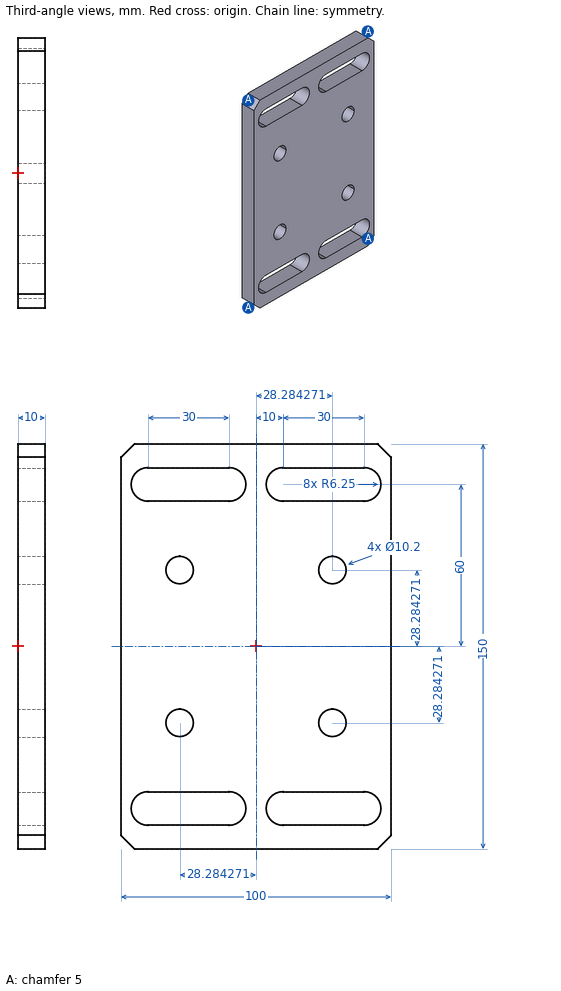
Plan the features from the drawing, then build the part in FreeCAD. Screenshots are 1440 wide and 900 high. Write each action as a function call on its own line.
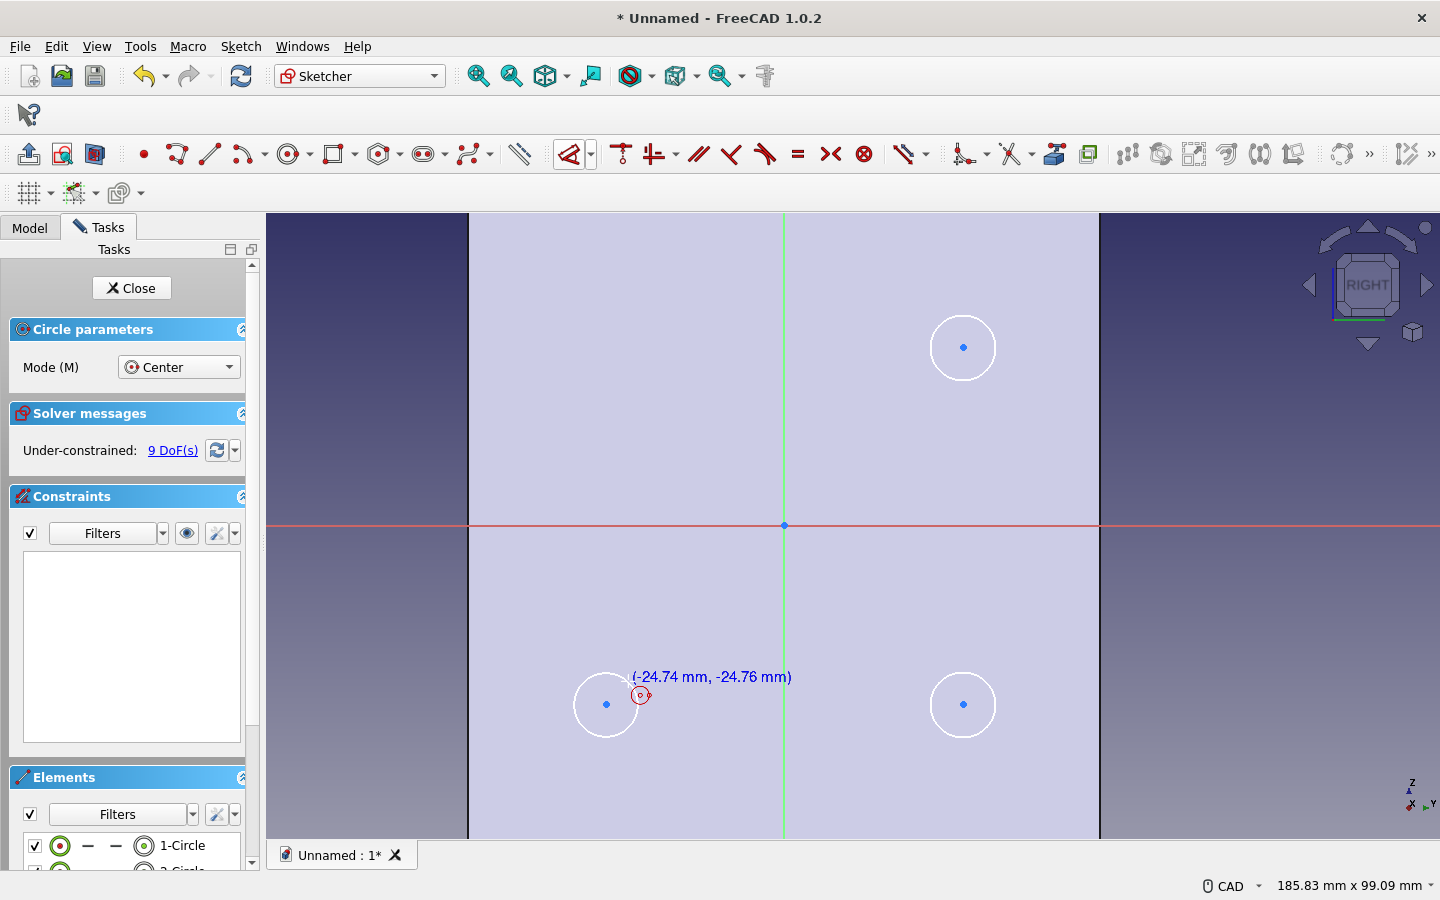
click(606, 347)
click(628, 324)
key(Escape)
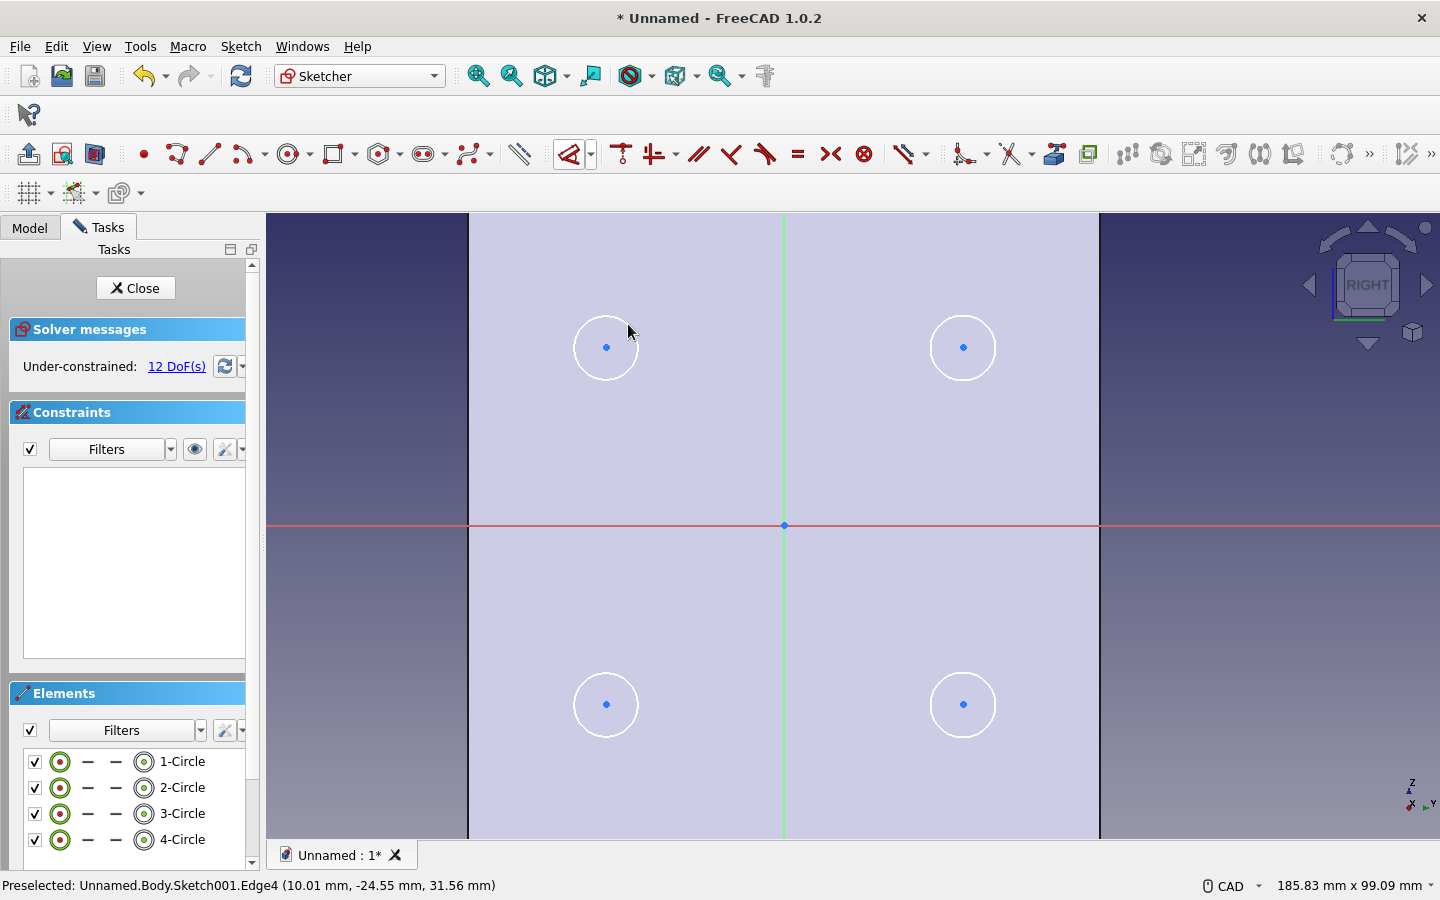
click(986, 325)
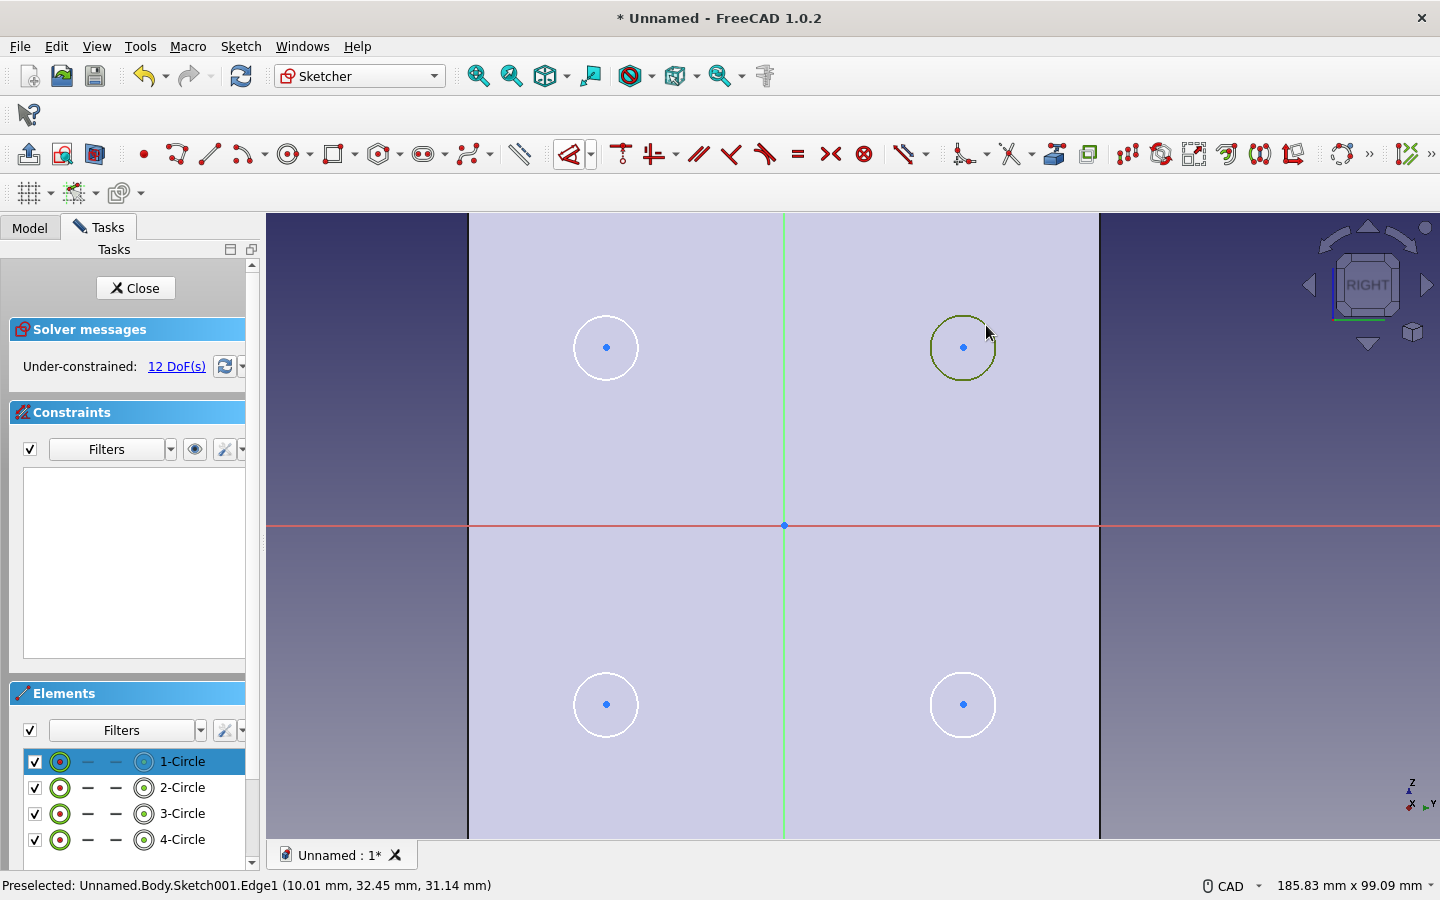
click(986, 682)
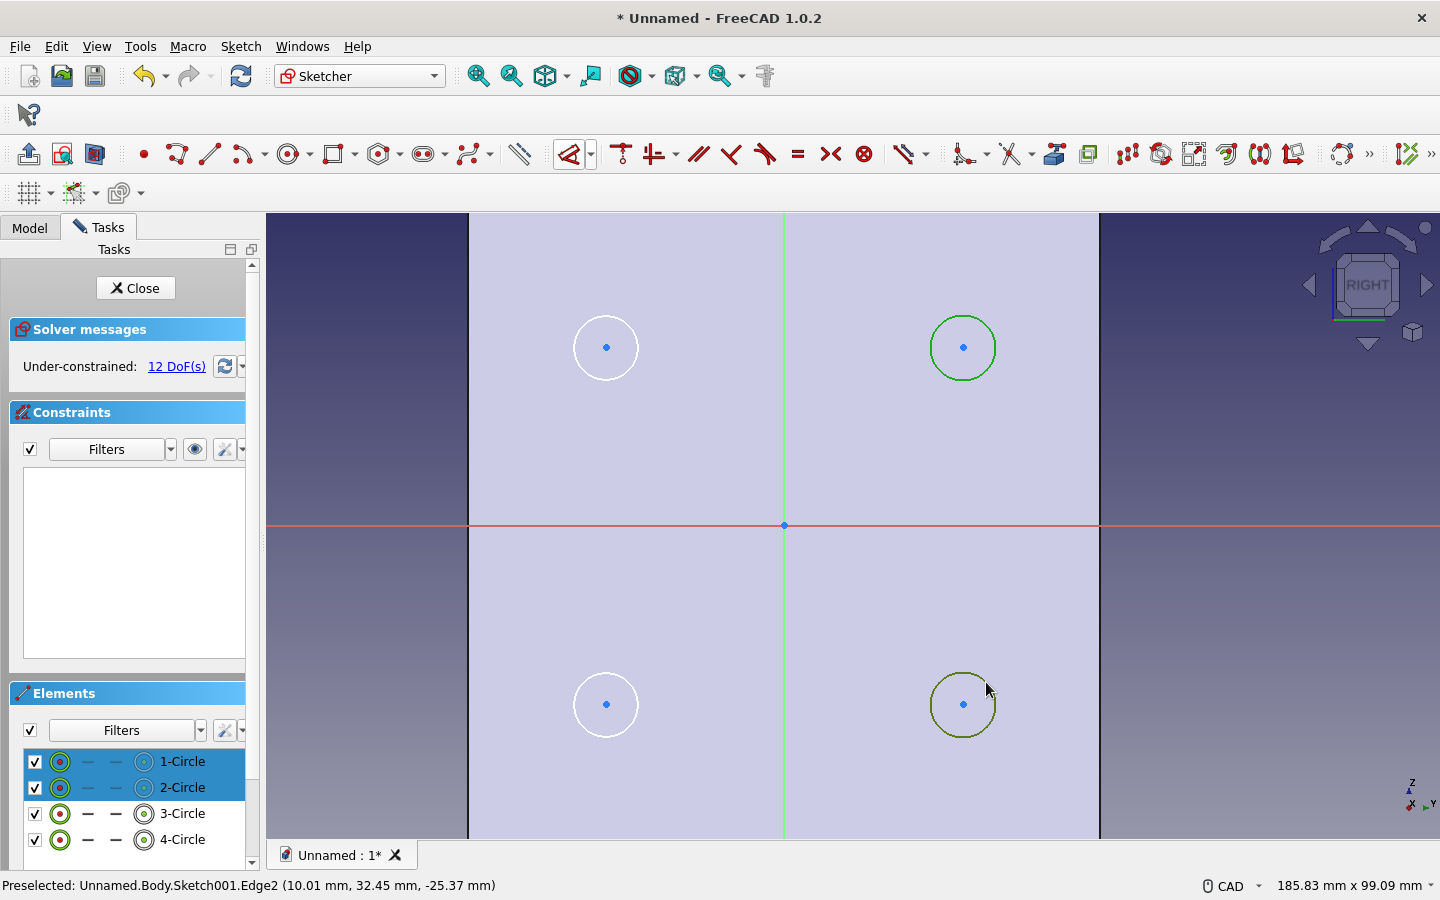
click(628, 682)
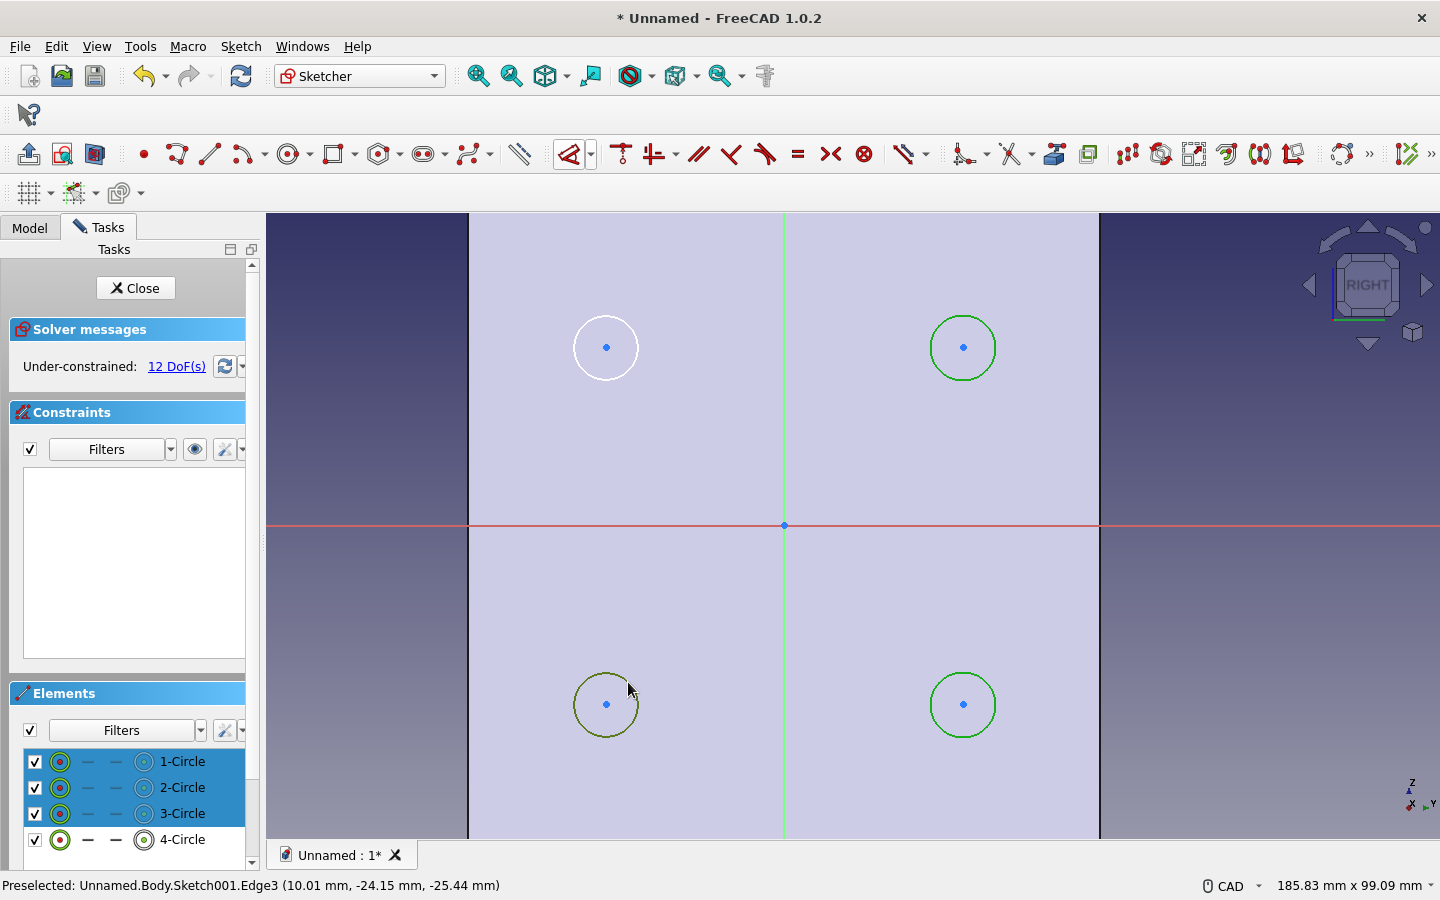
click(628, 325)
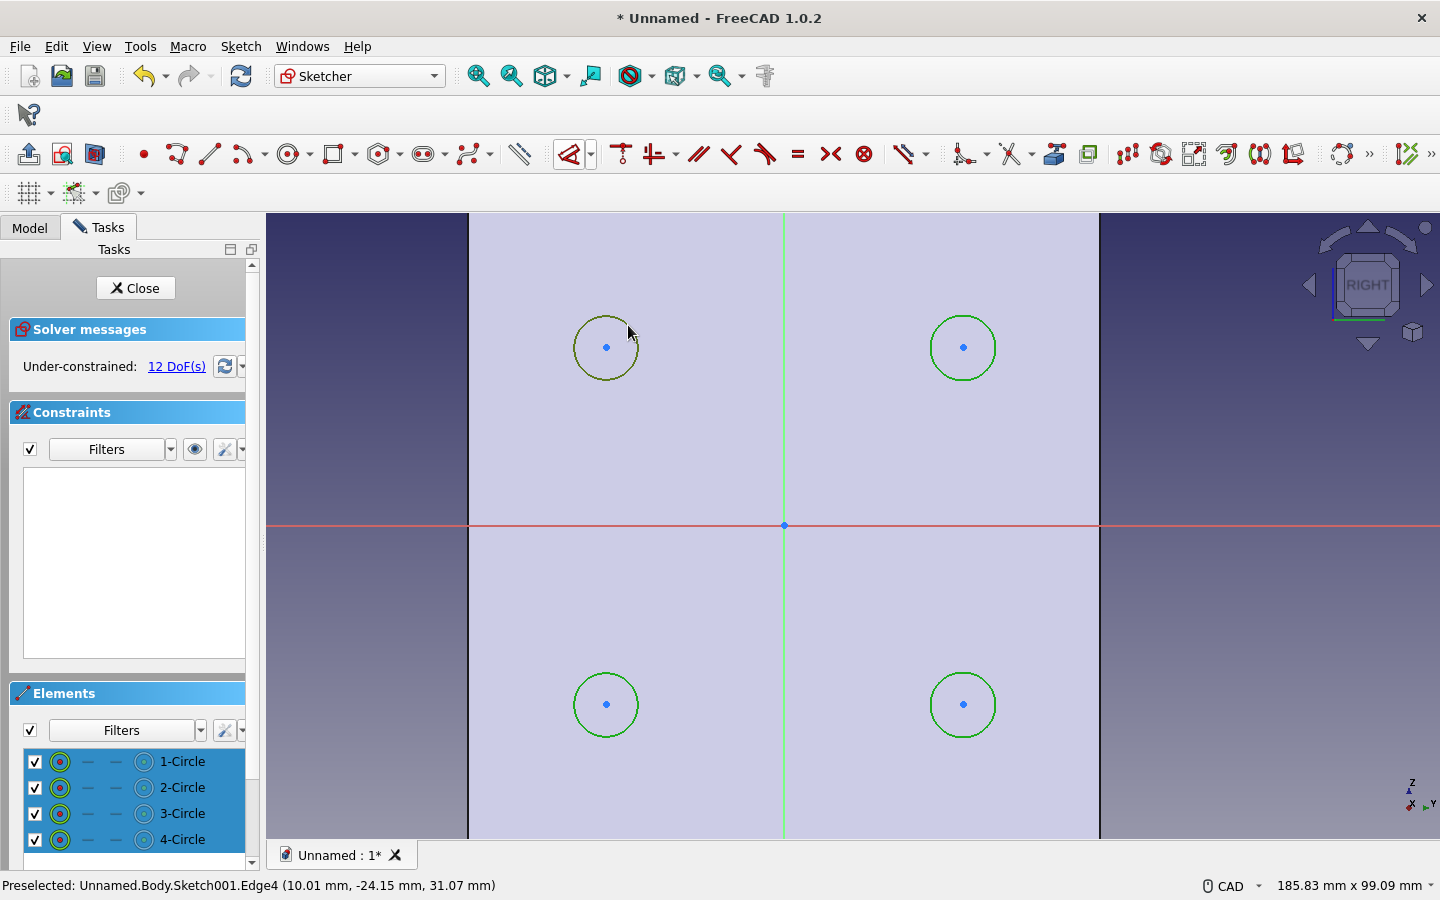
key(e)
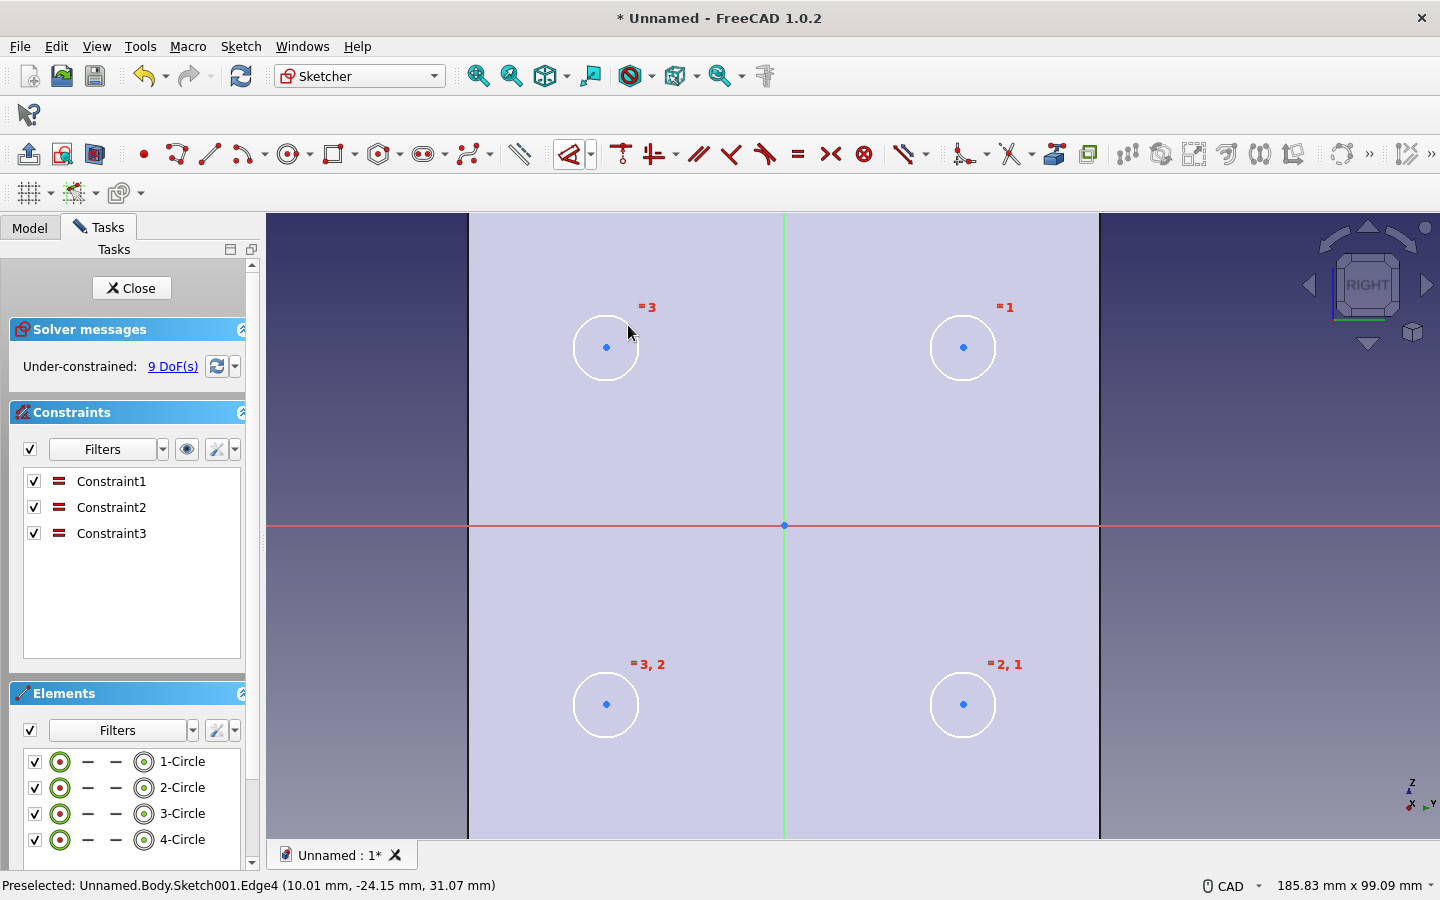
click(963, 348)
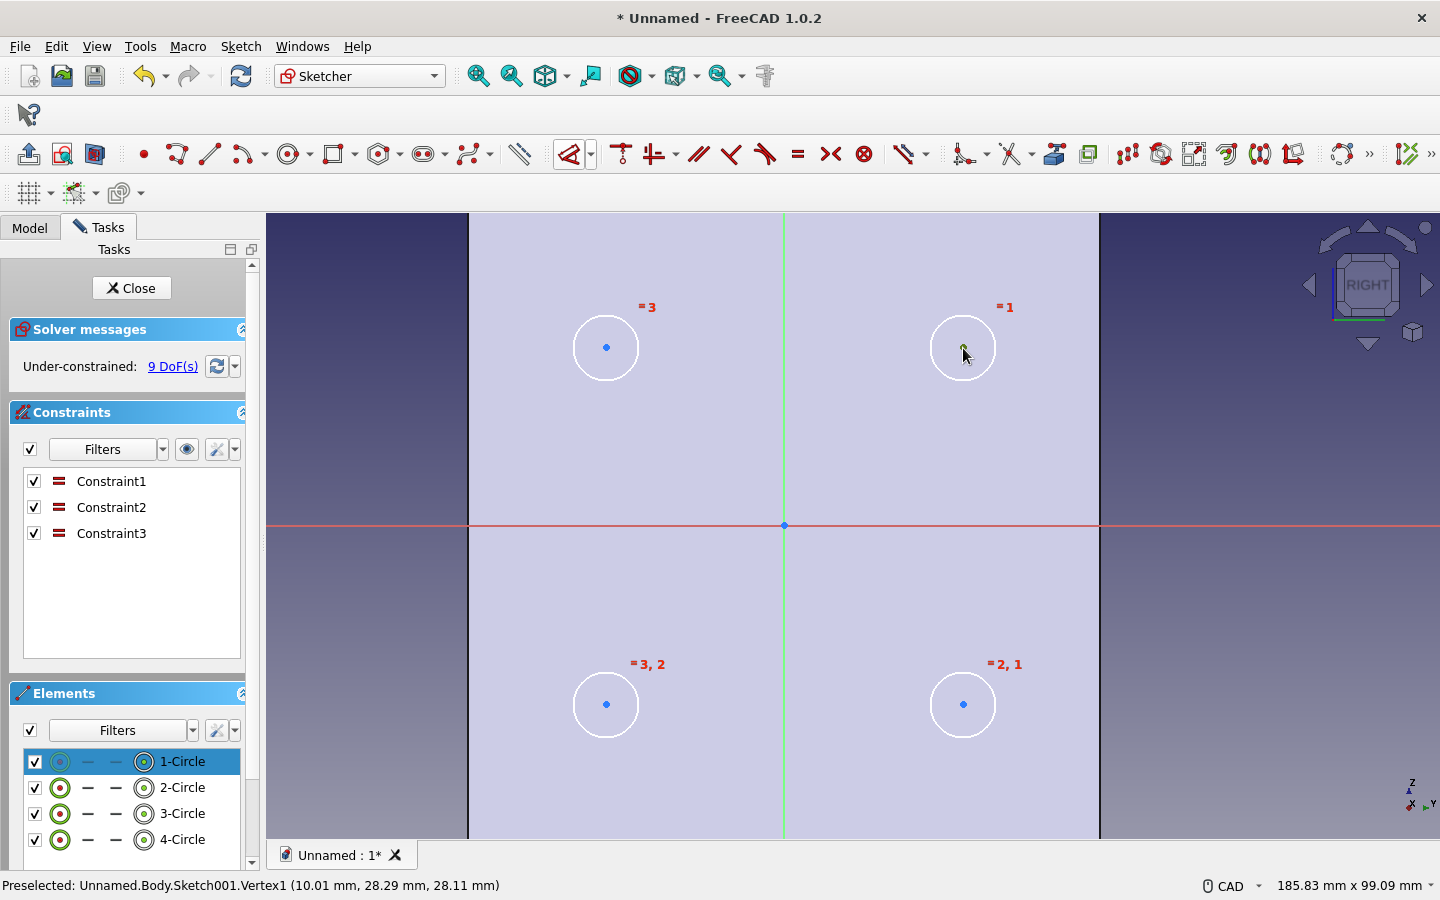
click(963, 705)